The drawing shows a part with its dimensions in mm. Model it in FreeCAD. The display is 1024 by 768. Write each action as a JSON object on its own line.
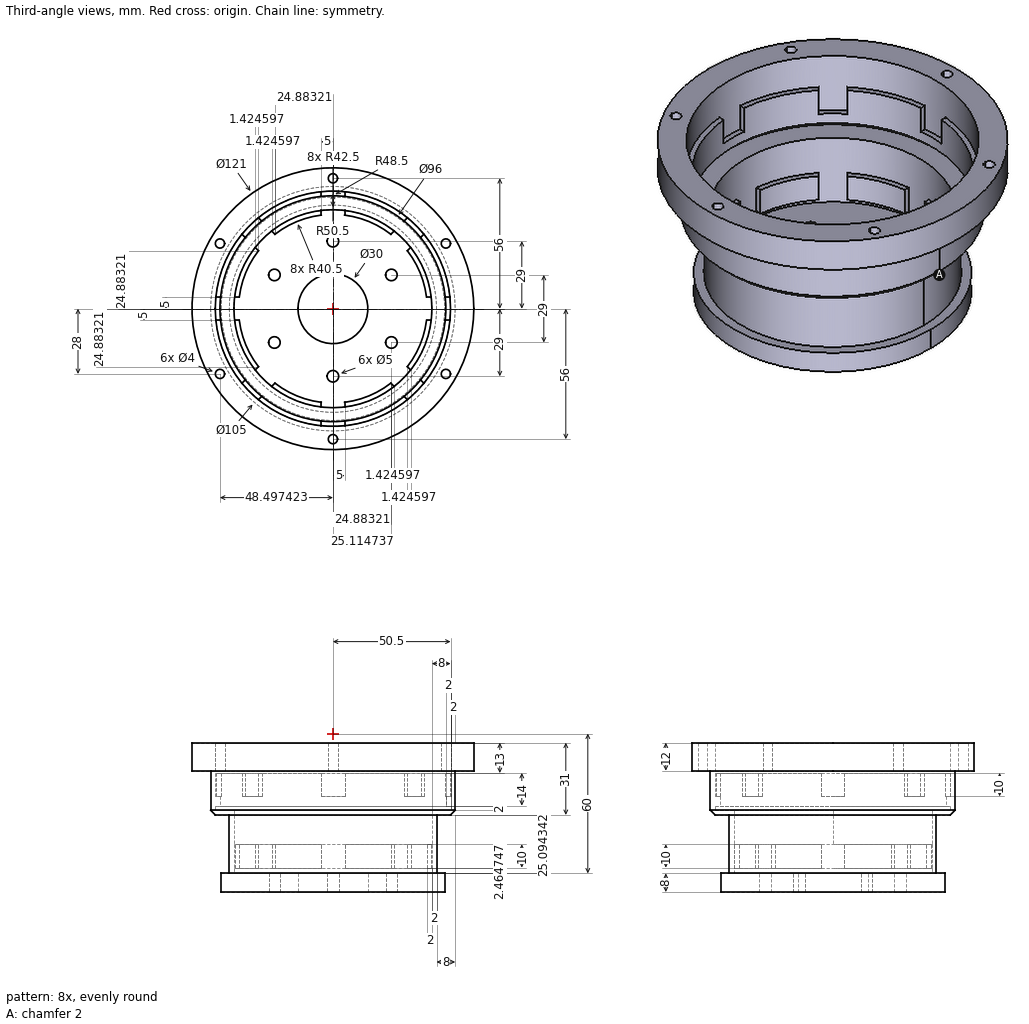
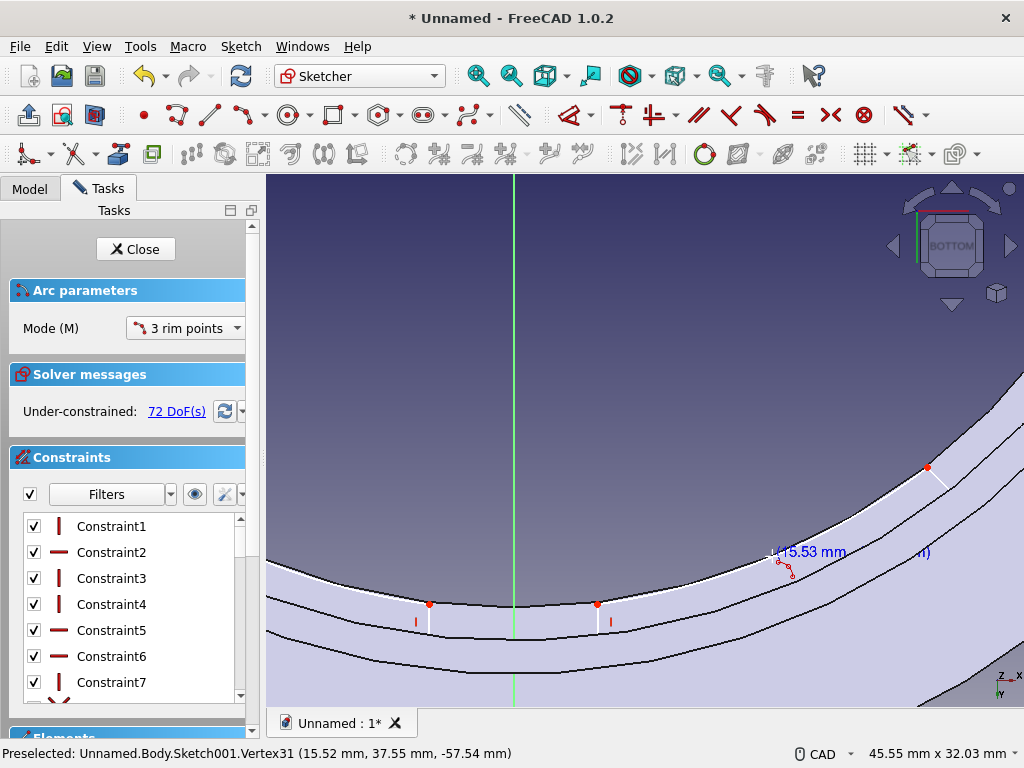
{"action": "left_click", "coordinate": [598, 639]}
{"action": "left_click", "coordinate": [429, 639]}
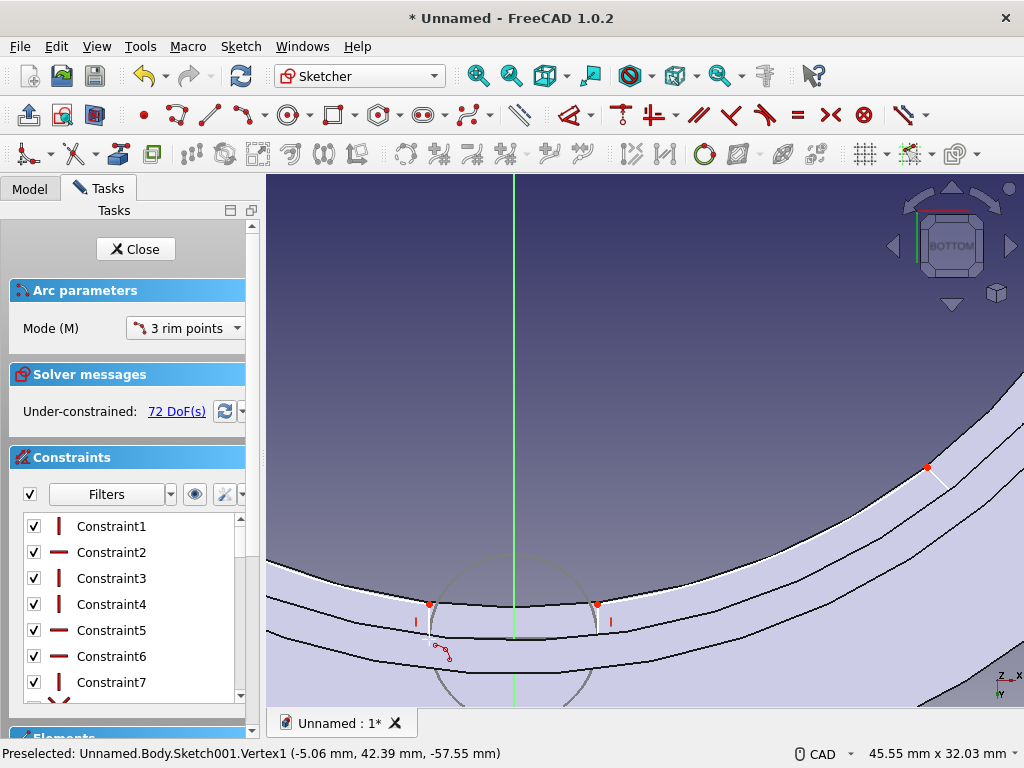
{"action": "scroll", "coordinate": [497, 641], "scroll_direction": "up", "scroll_amount": 7}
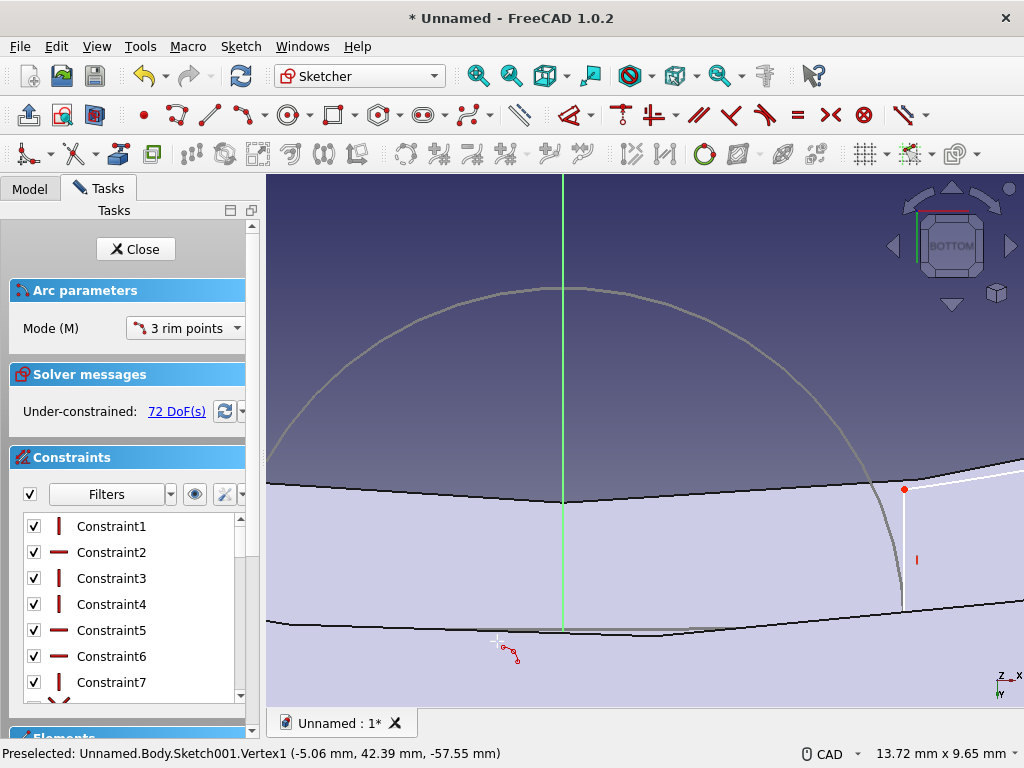
{"action": "left_click", "coordinate": [496, 637]}
{"action": "key", "text": "Escape"}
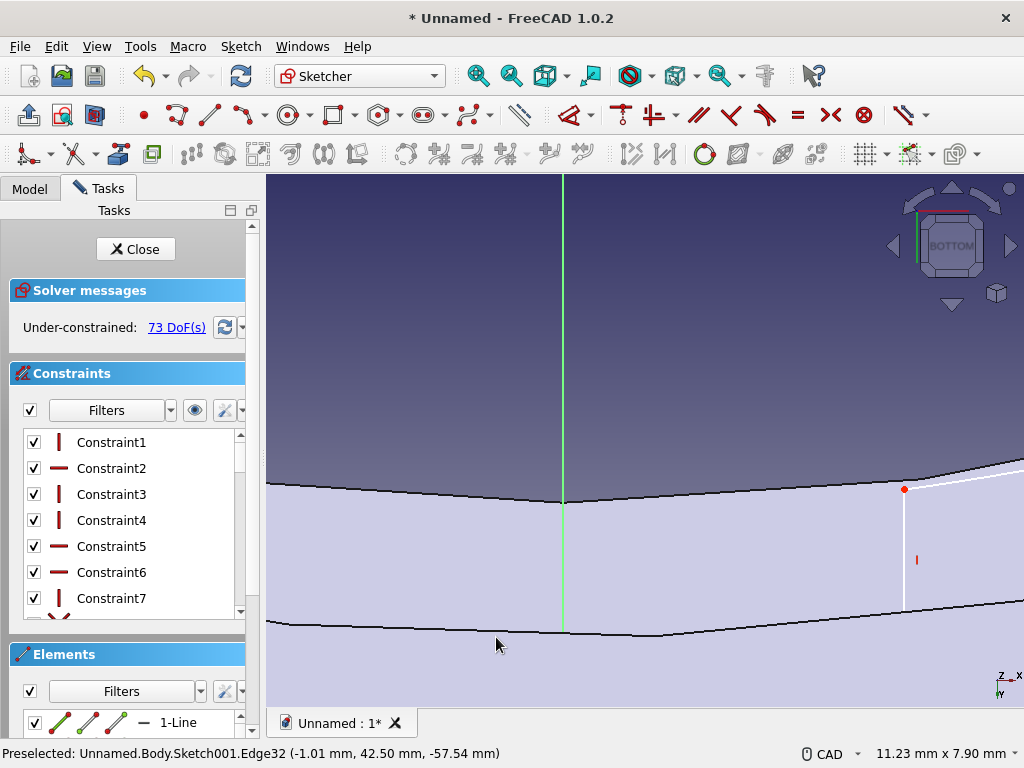
{"action": "scroll", "coordinate": [577, 613], "scroll_direction": "down", "scroll_amount": 14}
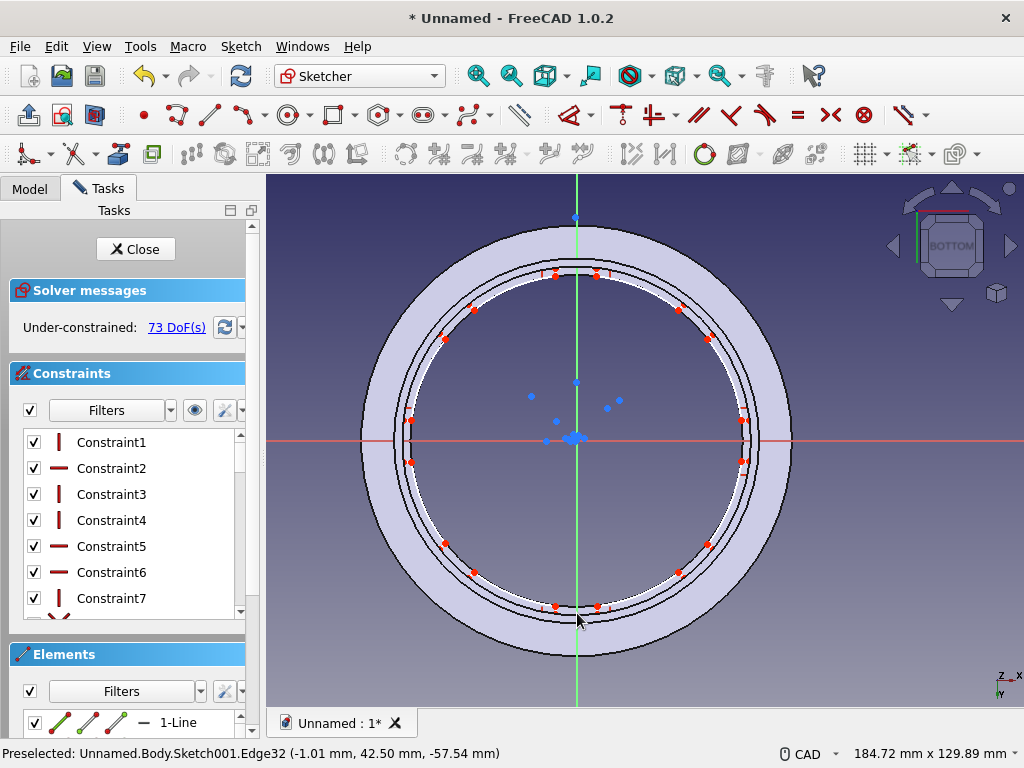
{"action": "scroll", "coordinate": [409, 463], "scroll_direction": "up", "scroll_amount": 9}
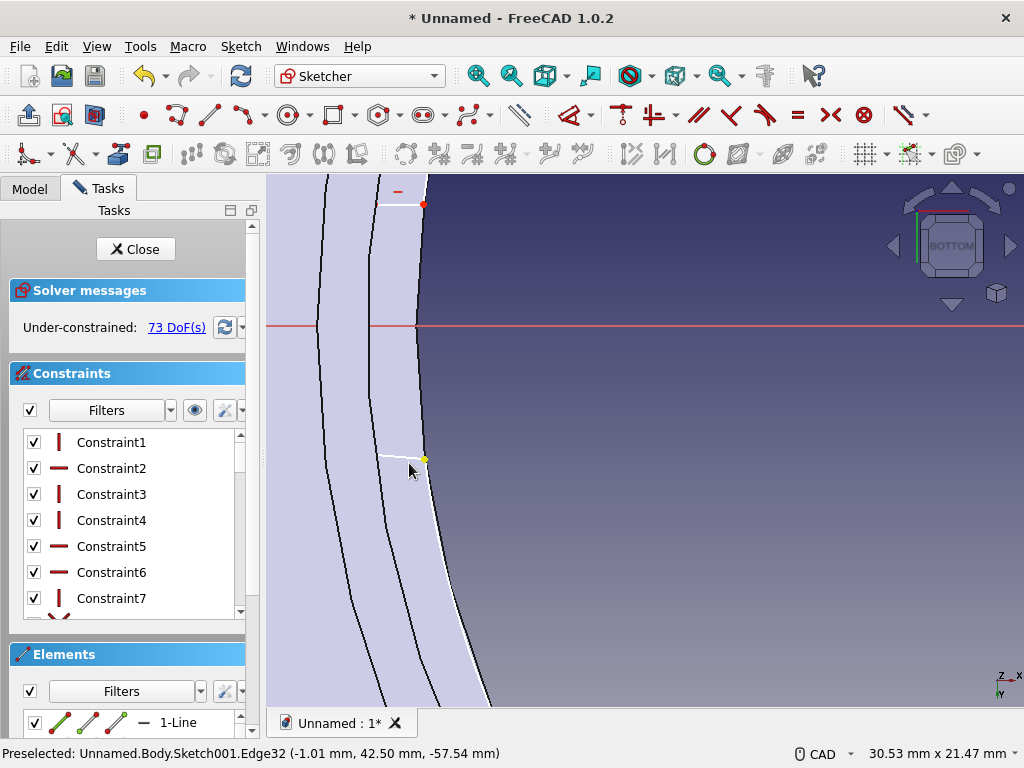
{"action": "left_click", "coordinate": [410, 458]}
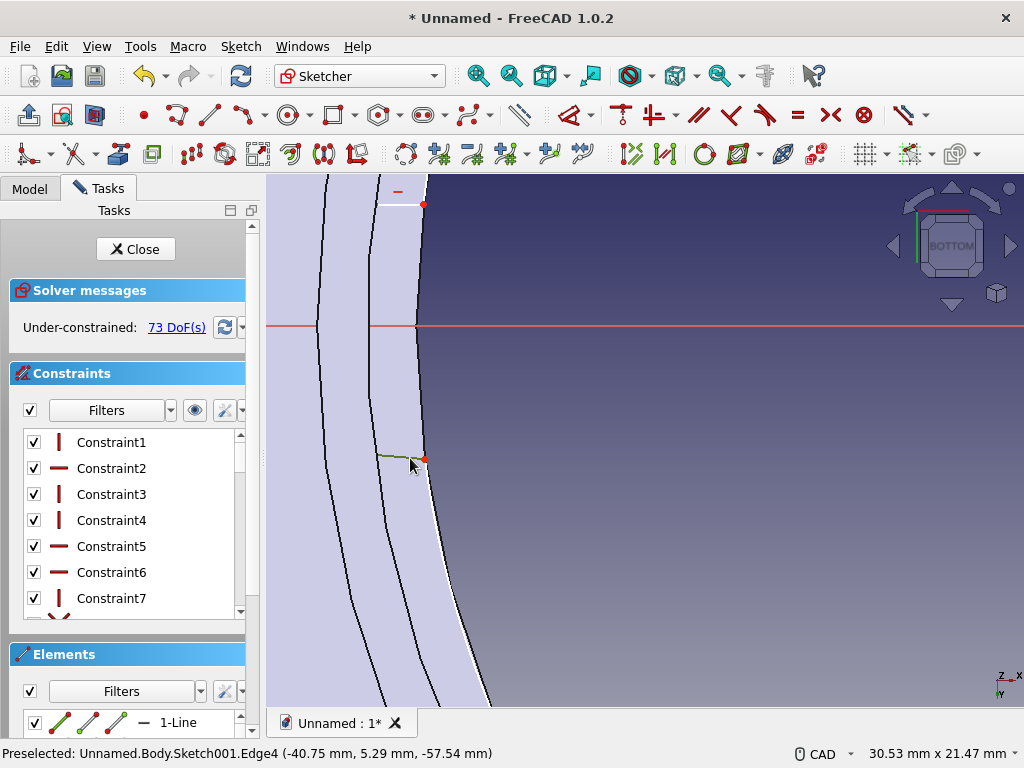
{"action": "key", "text": "h"}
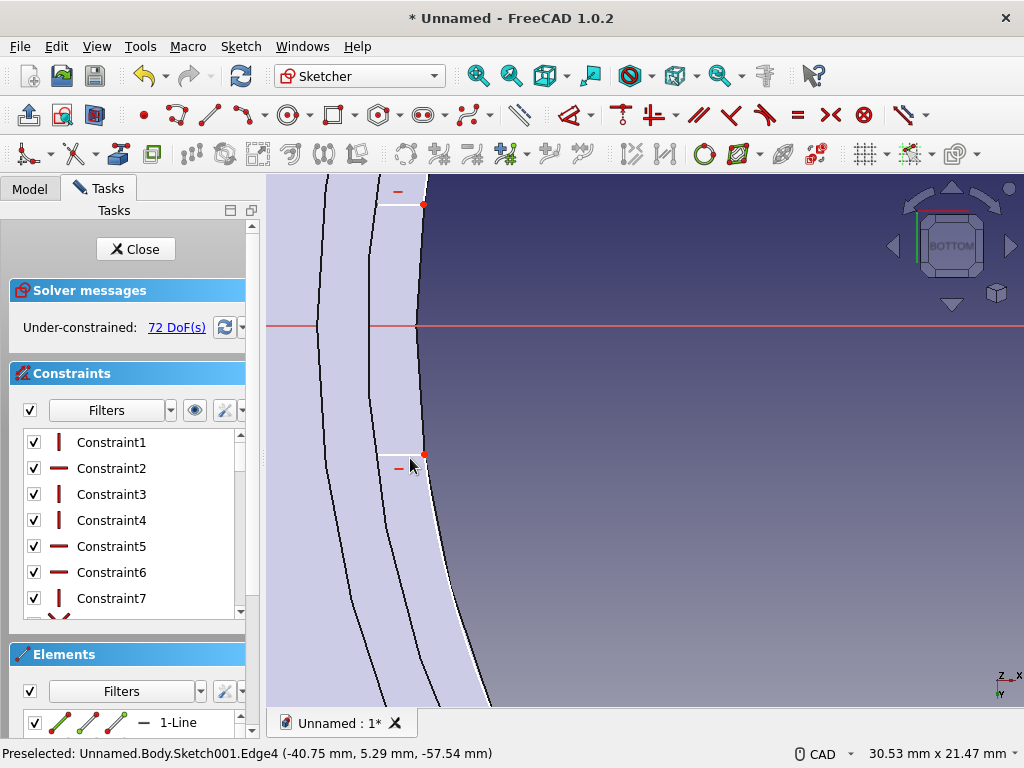
{"action": "scroll", "coordinate": [409, 463], "scroll_direction": "down", "scroll_amount": 9}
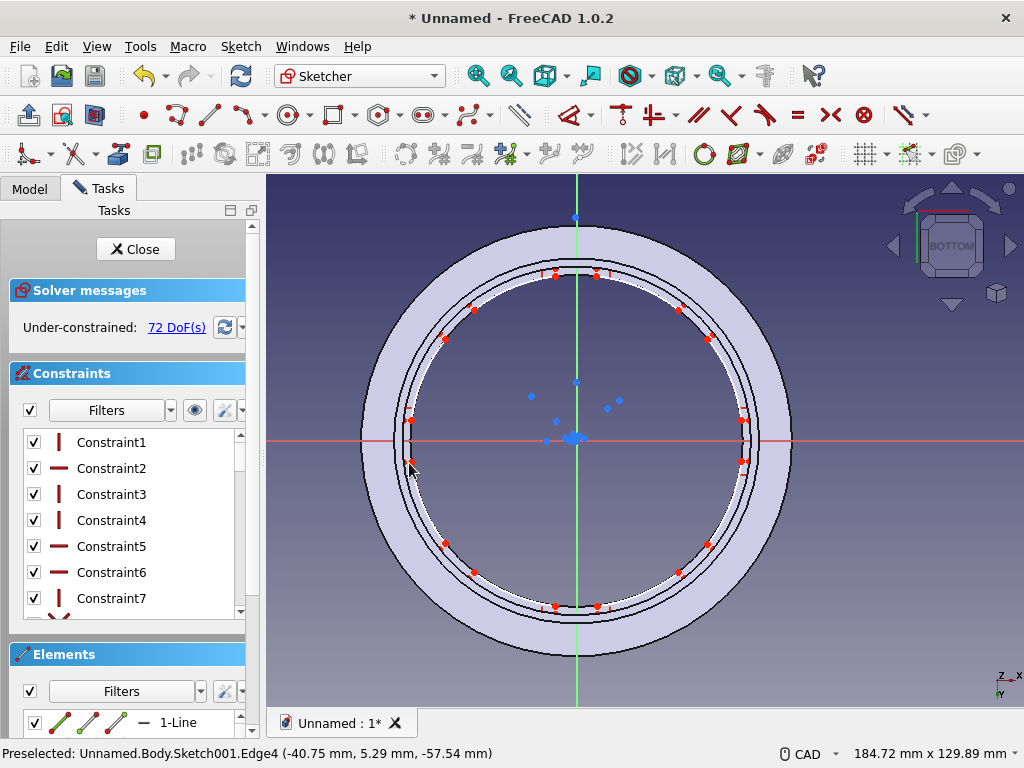
{"action": "left_click", "coordinate": [497, 587]}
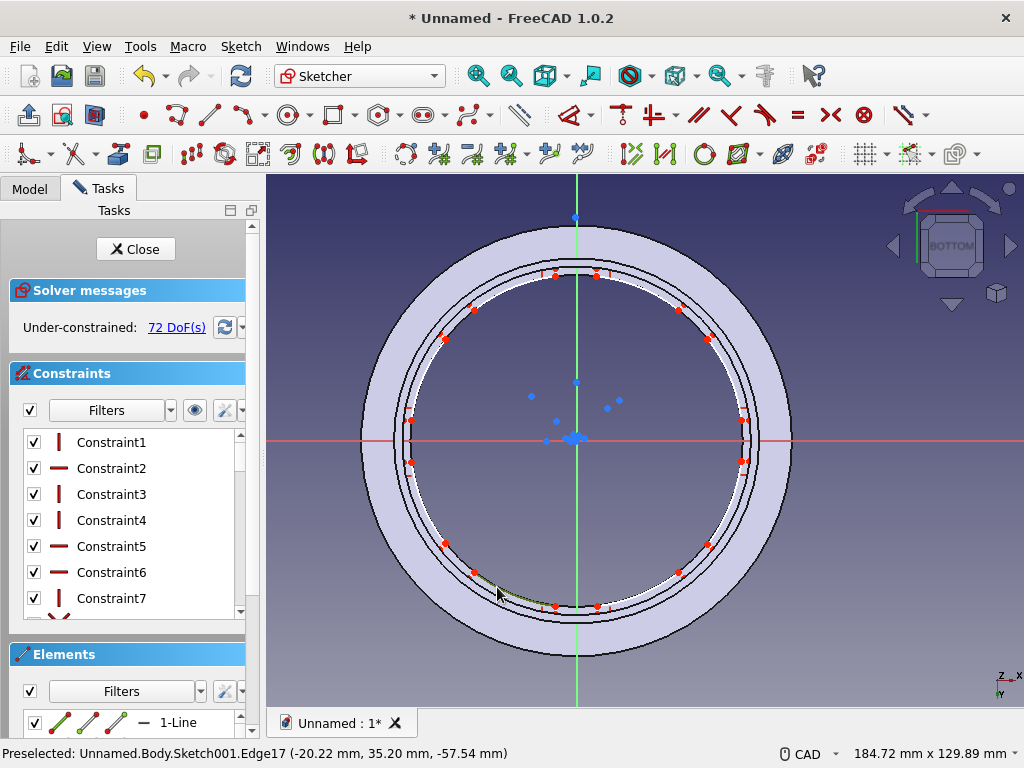
{"action": "left_click", "coordinate": [448, 558]}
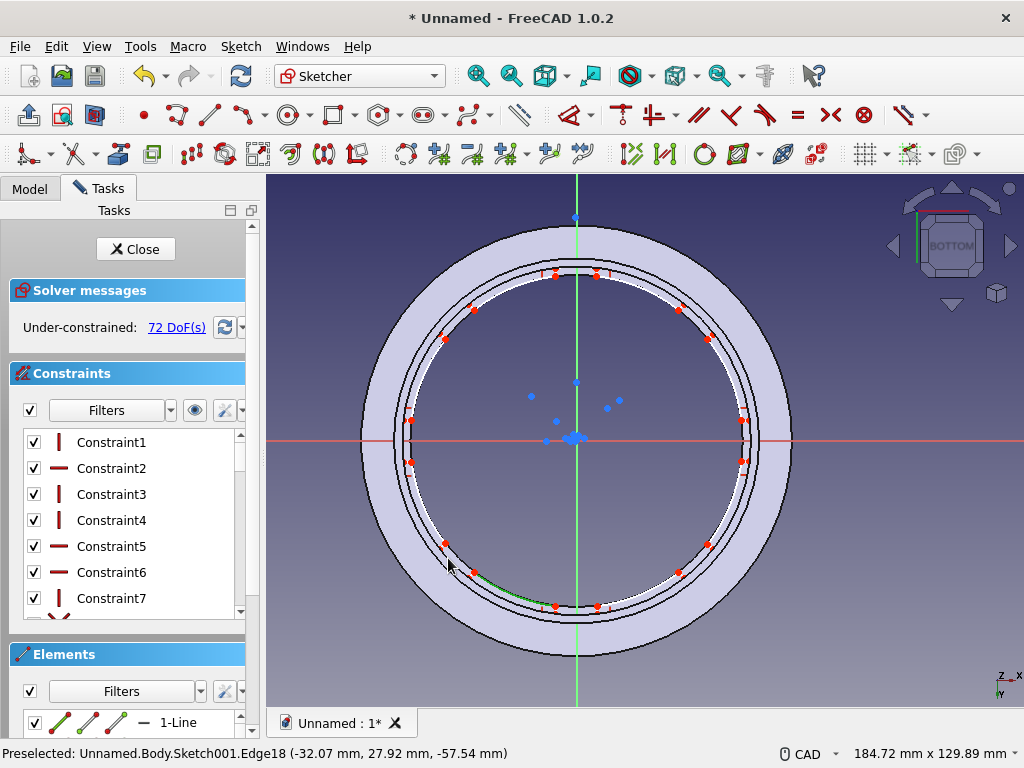
{"action": "key", "text": "c"}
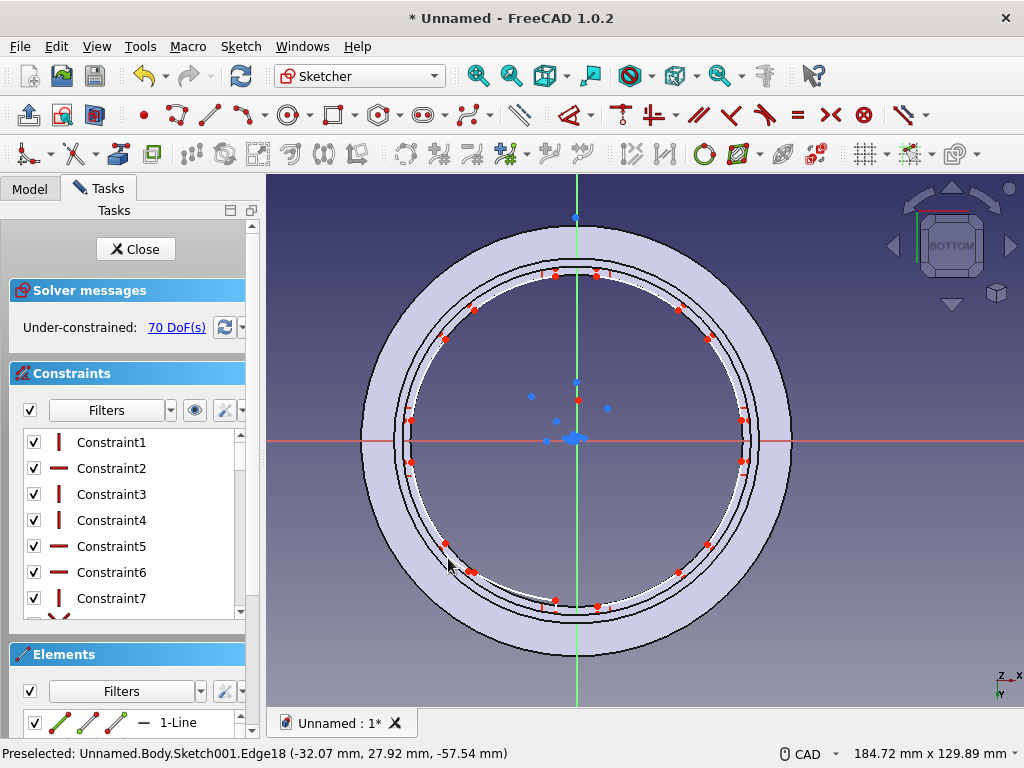
{"action": "left_click", "coordinate": [497, 585]}